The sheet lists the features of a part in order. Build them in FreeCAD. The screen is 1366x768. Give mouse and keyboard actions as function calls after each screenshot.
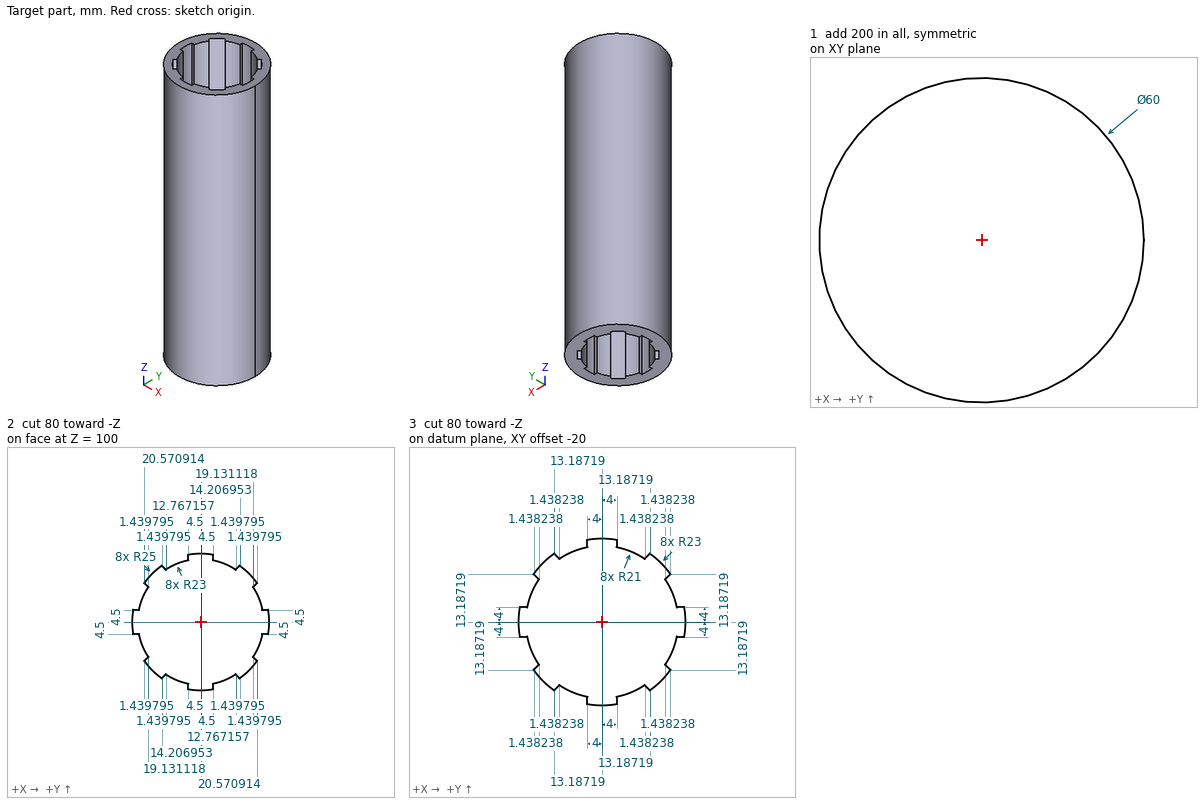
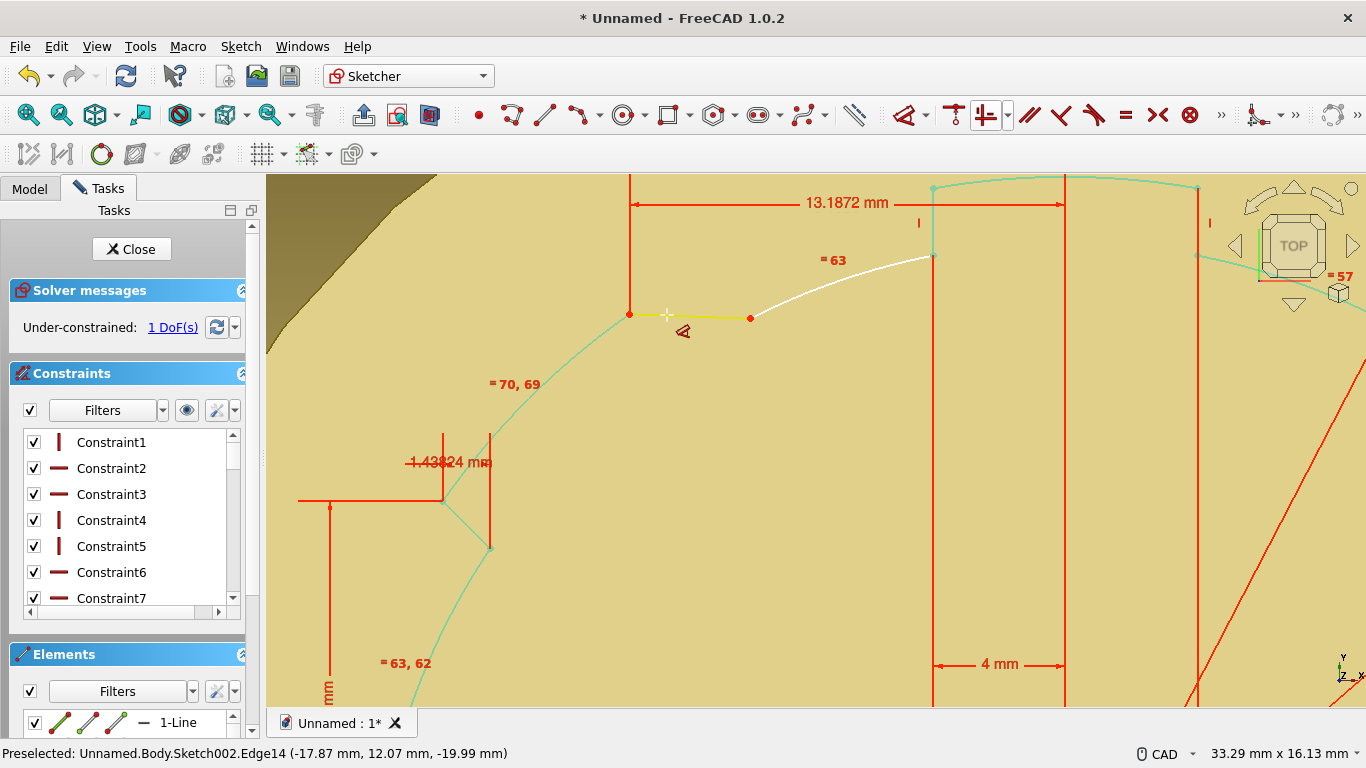
click(666, 316)
click(690, 280)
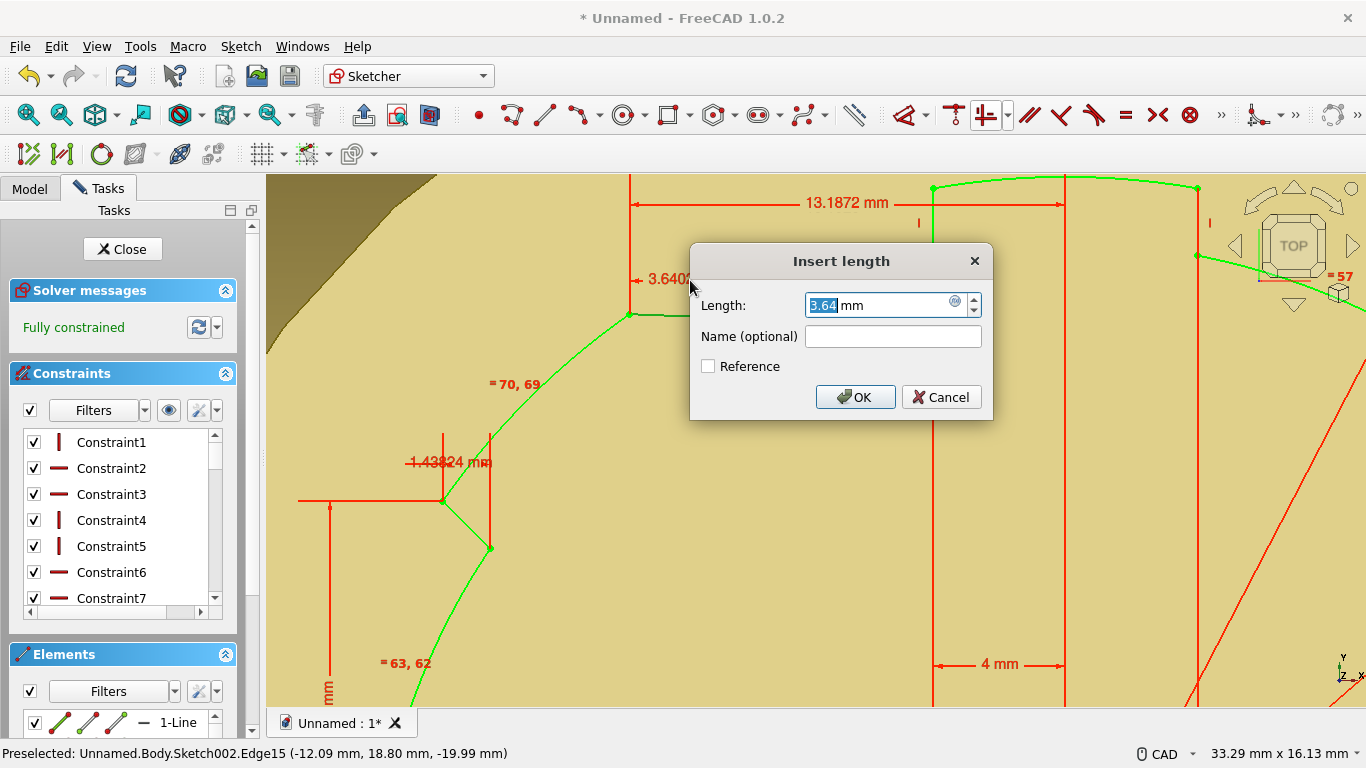
text(1.438238)
key(Return)
key(Escape)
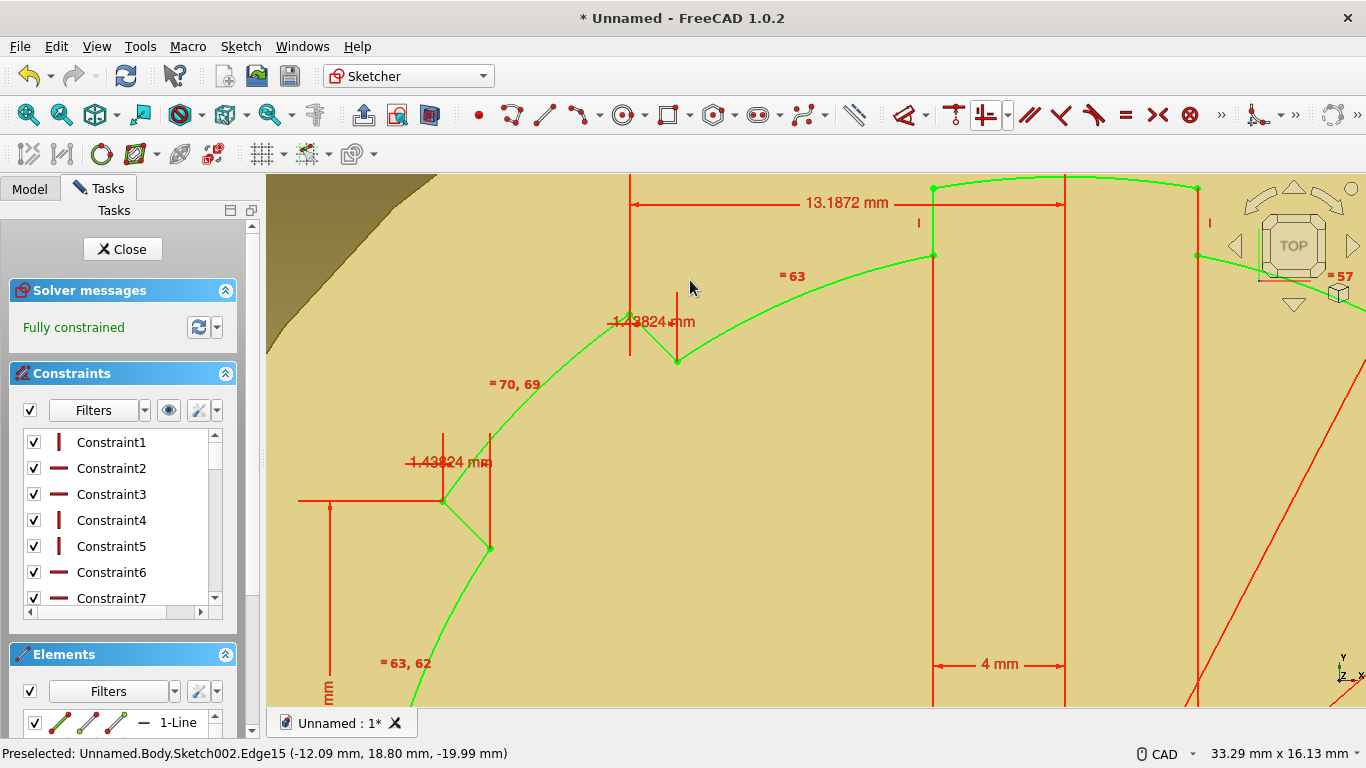
click(123, 249)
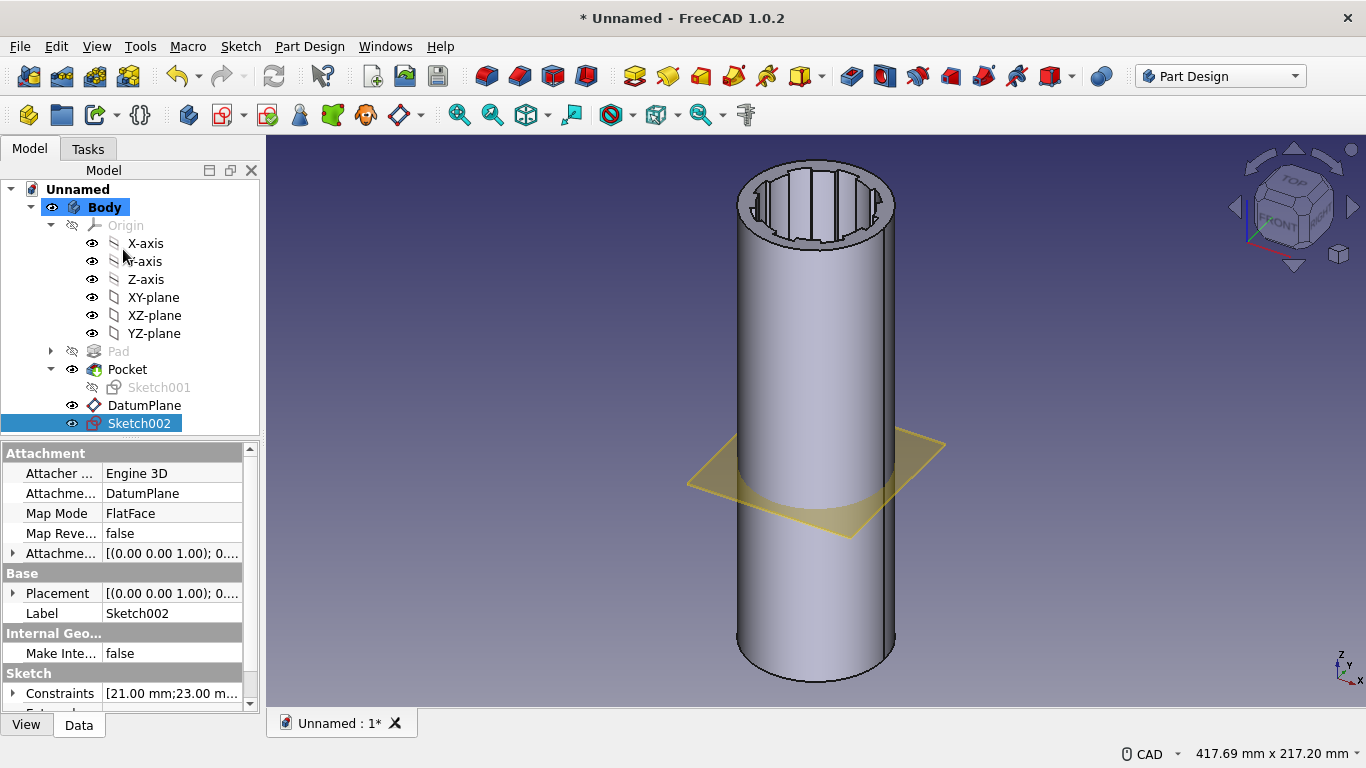
click(852, 76)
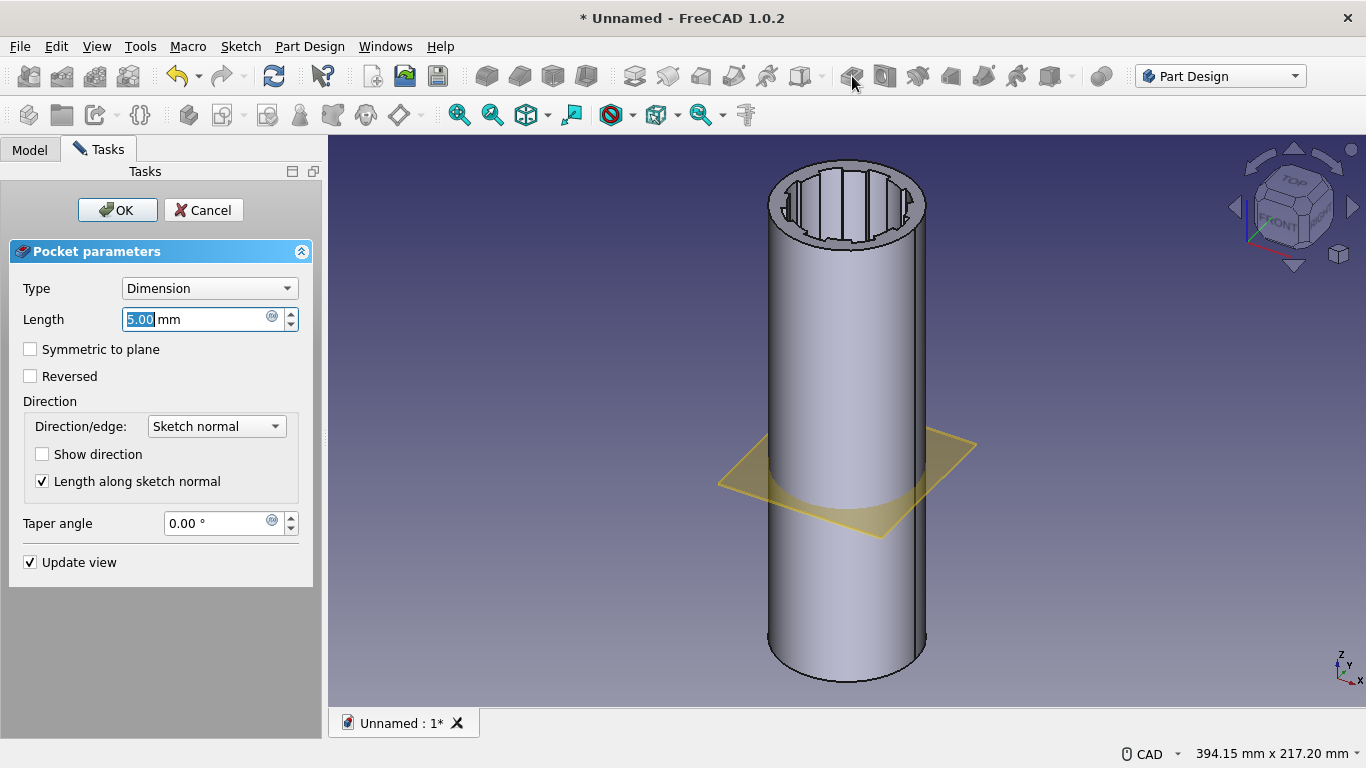
text(80)
key(Tab)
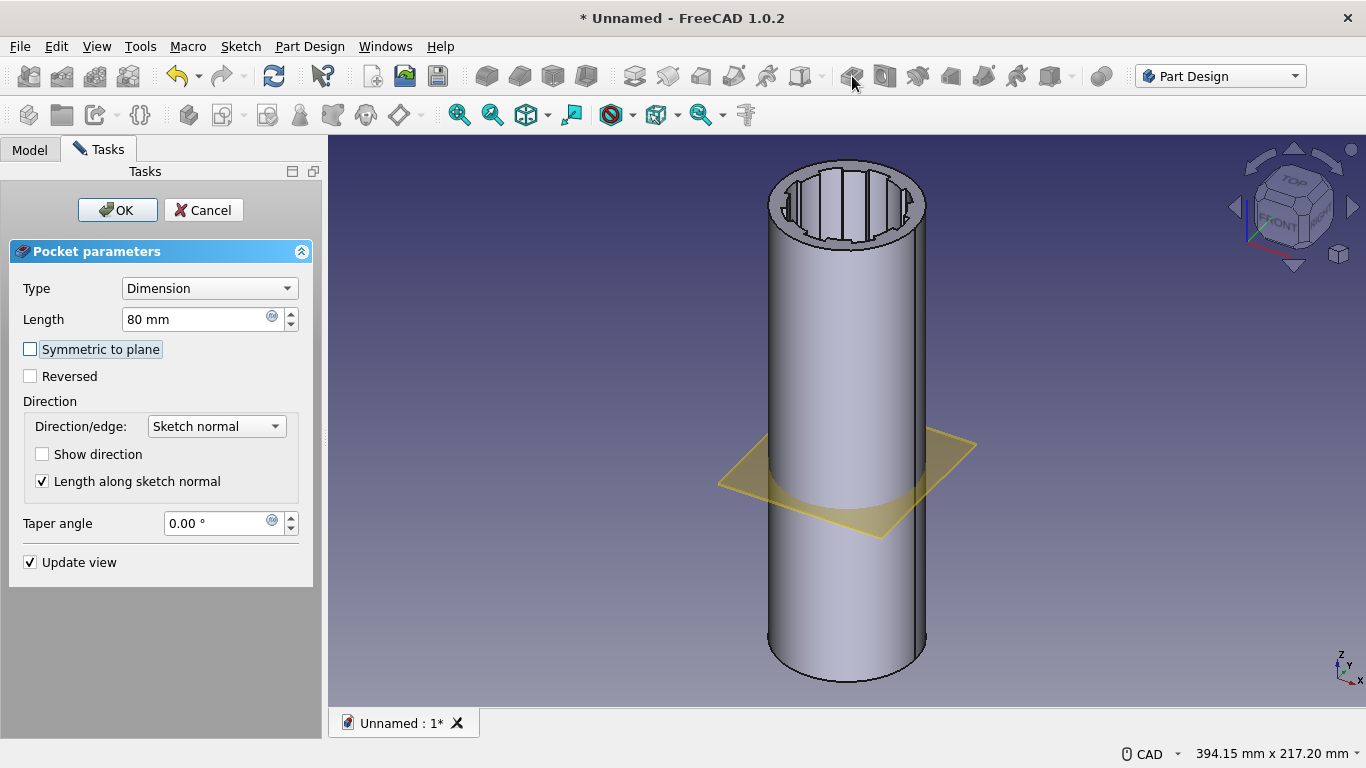
click(118, 210)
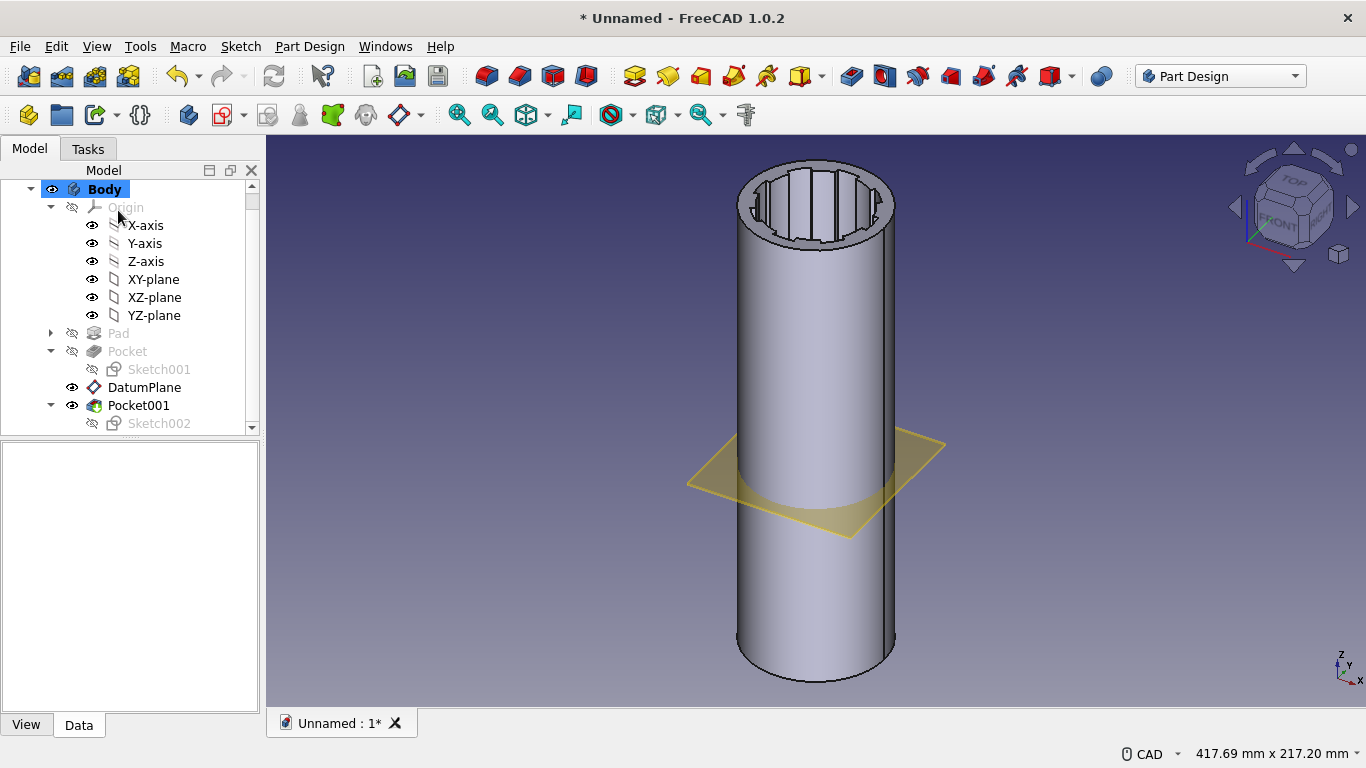
click(117, 387)
key(space)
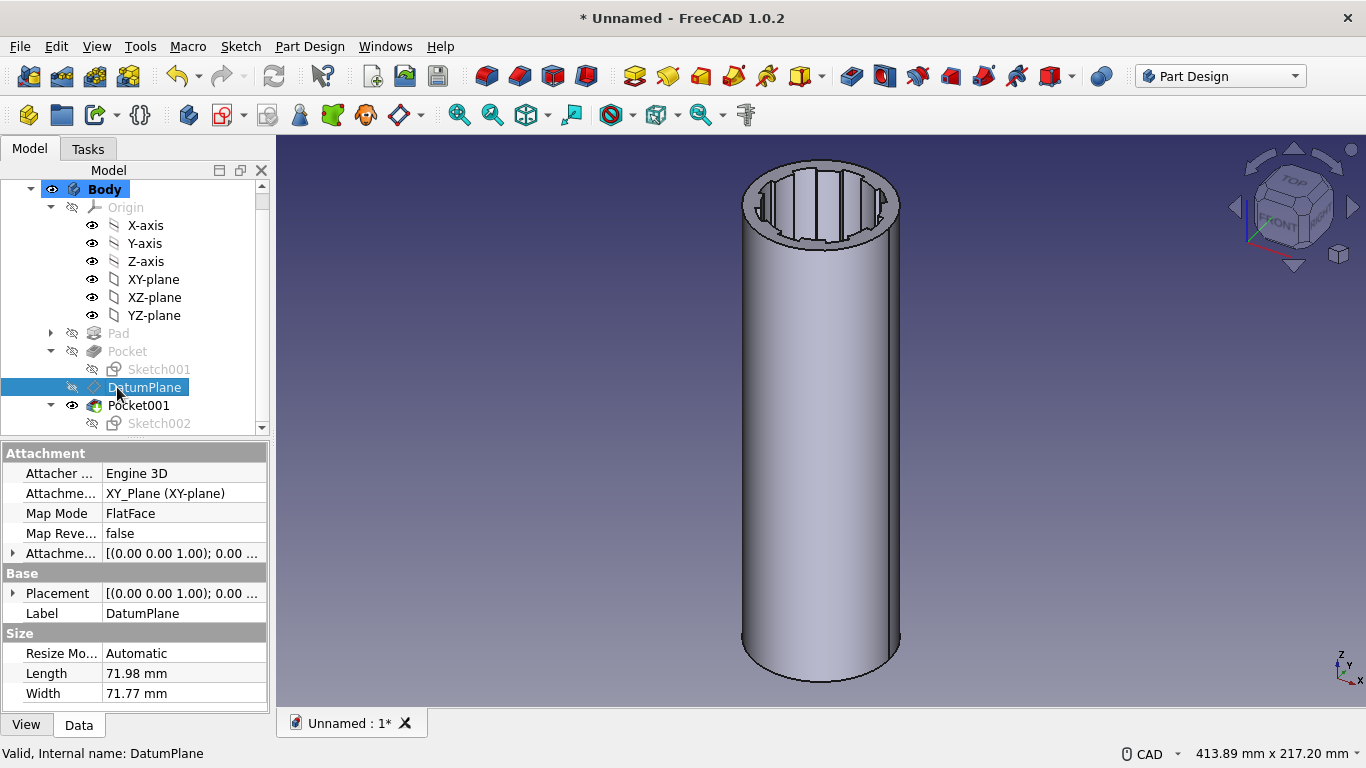
key(0)